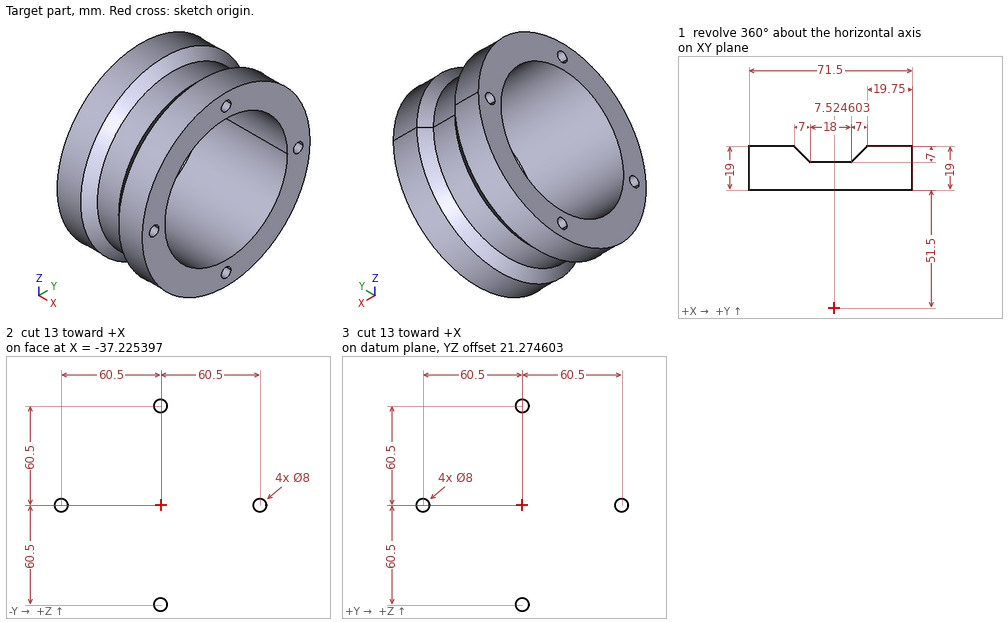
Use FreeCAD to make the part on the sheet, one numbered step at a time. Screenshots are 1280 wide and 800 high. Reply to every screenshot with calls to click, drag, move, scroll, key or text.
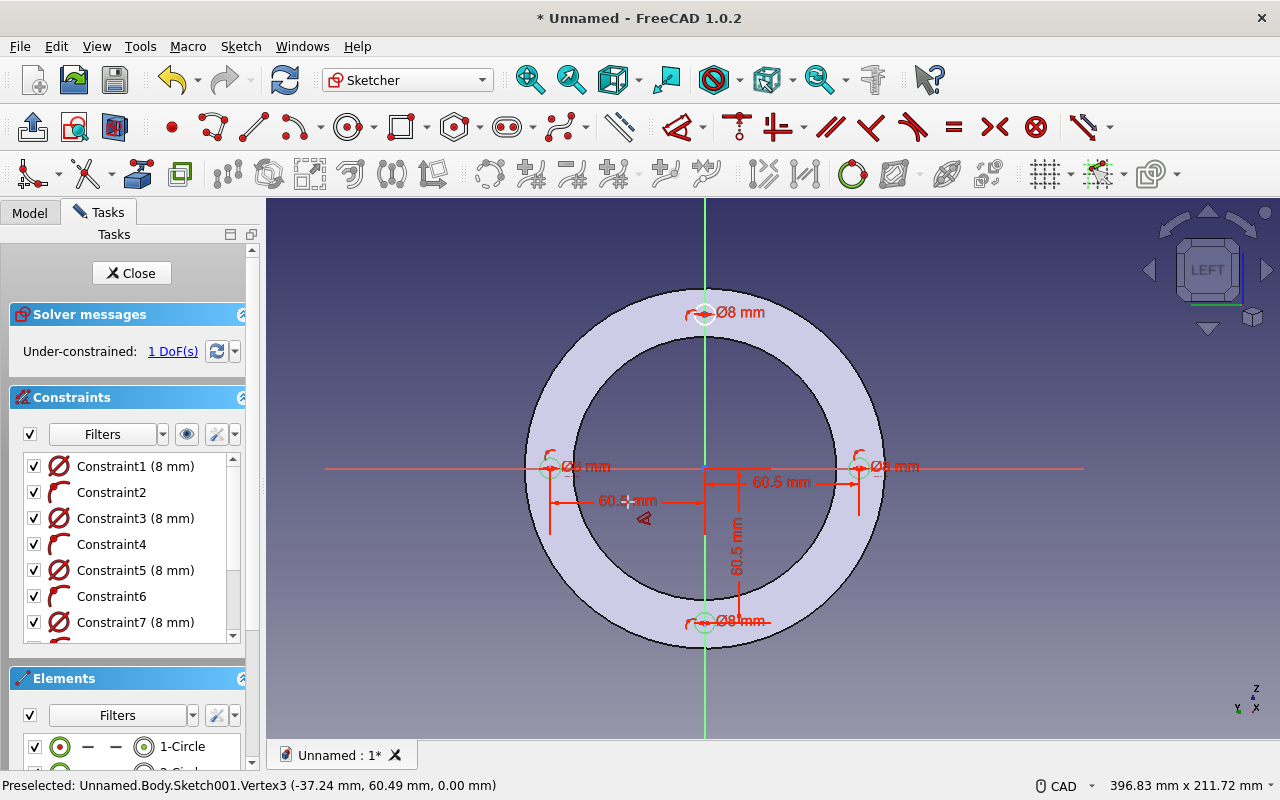
click(705, 314)
click(739, 391)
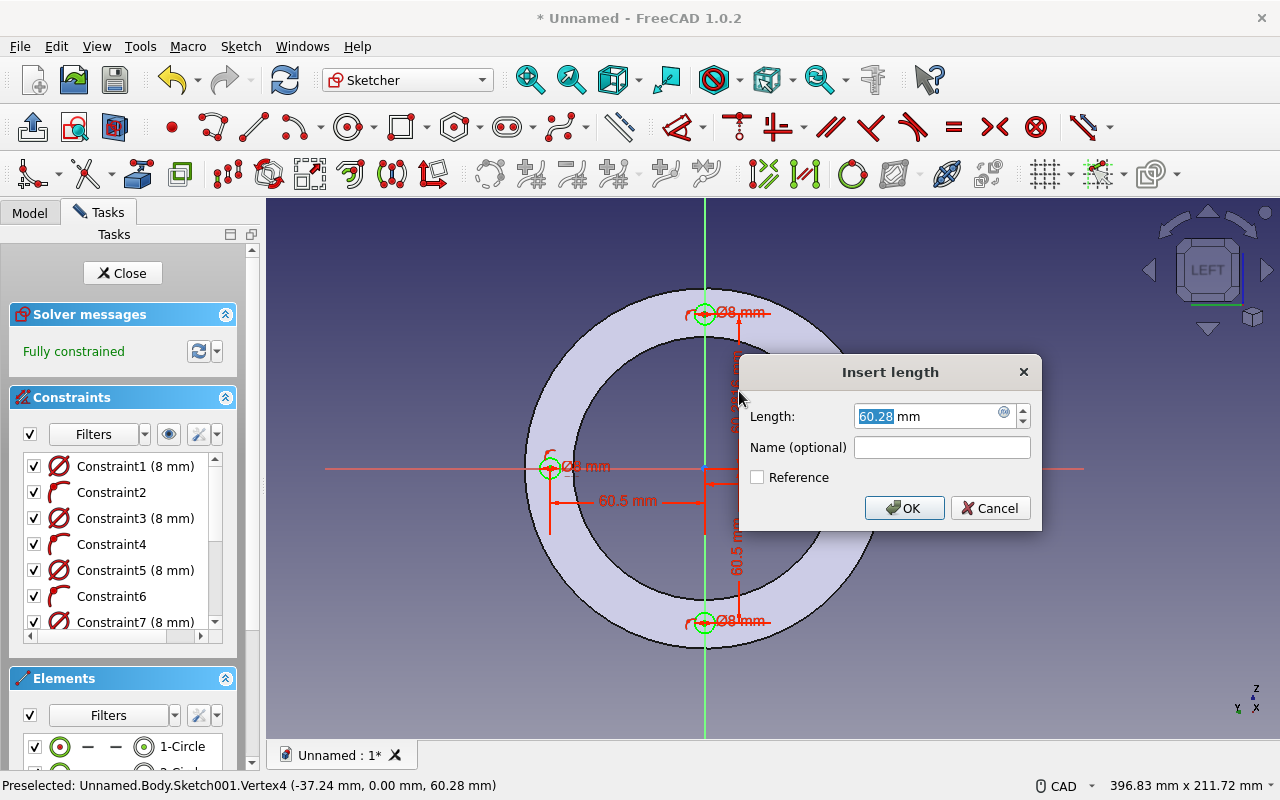
text(60.5)
key(Return)
key(Escape)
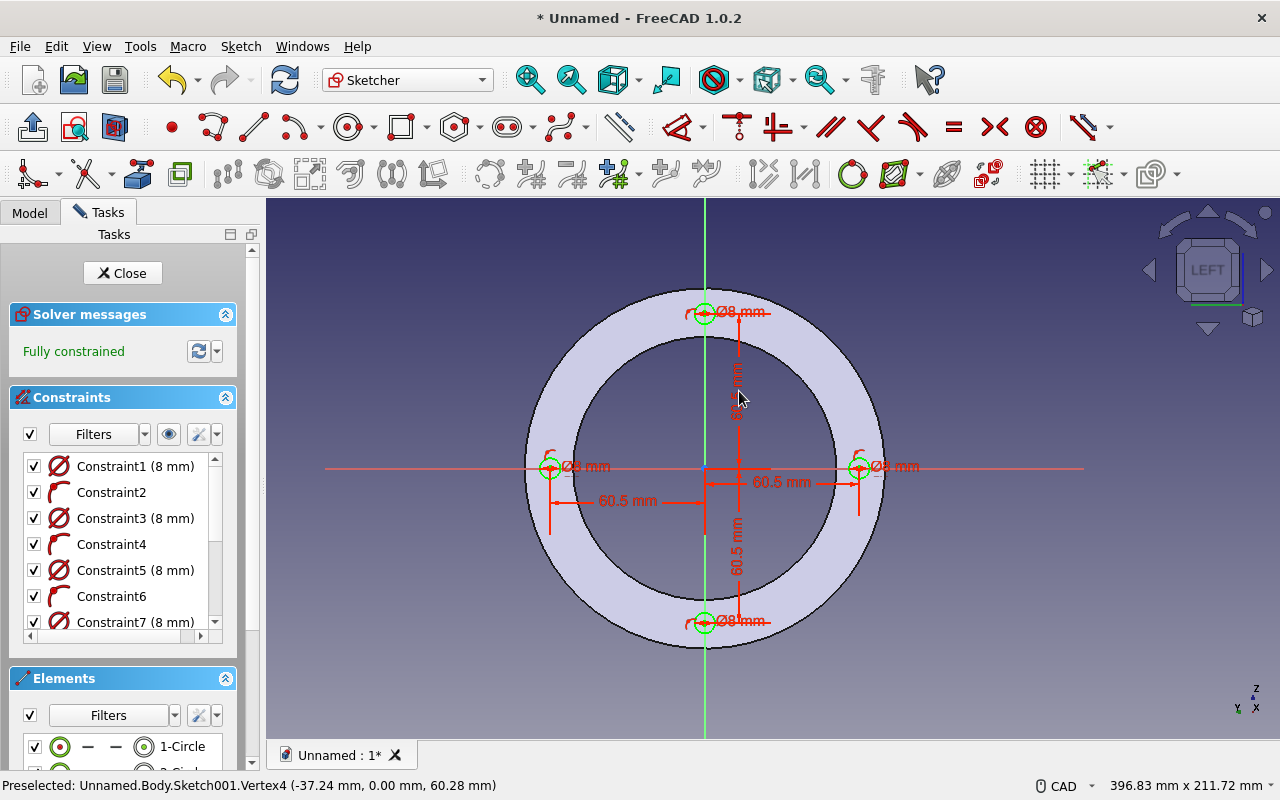
click(123, 273)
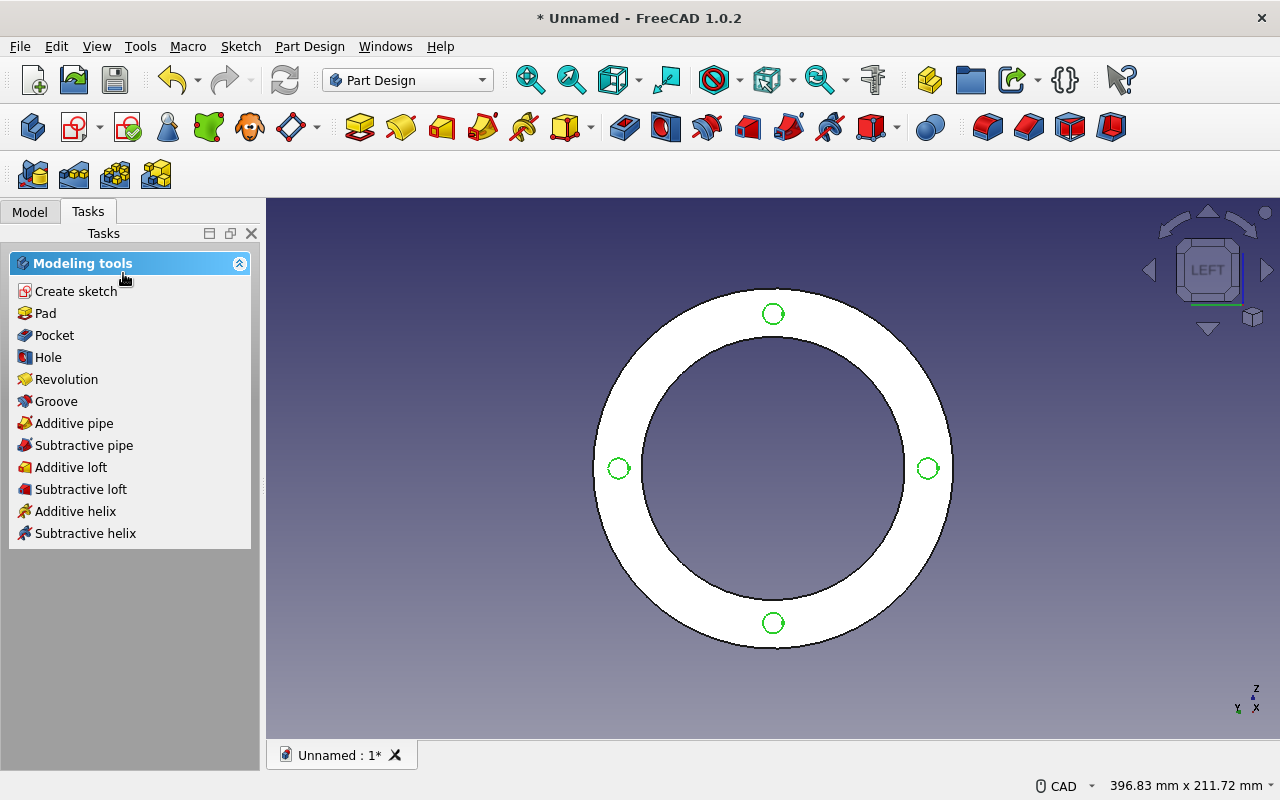
click(625, 128)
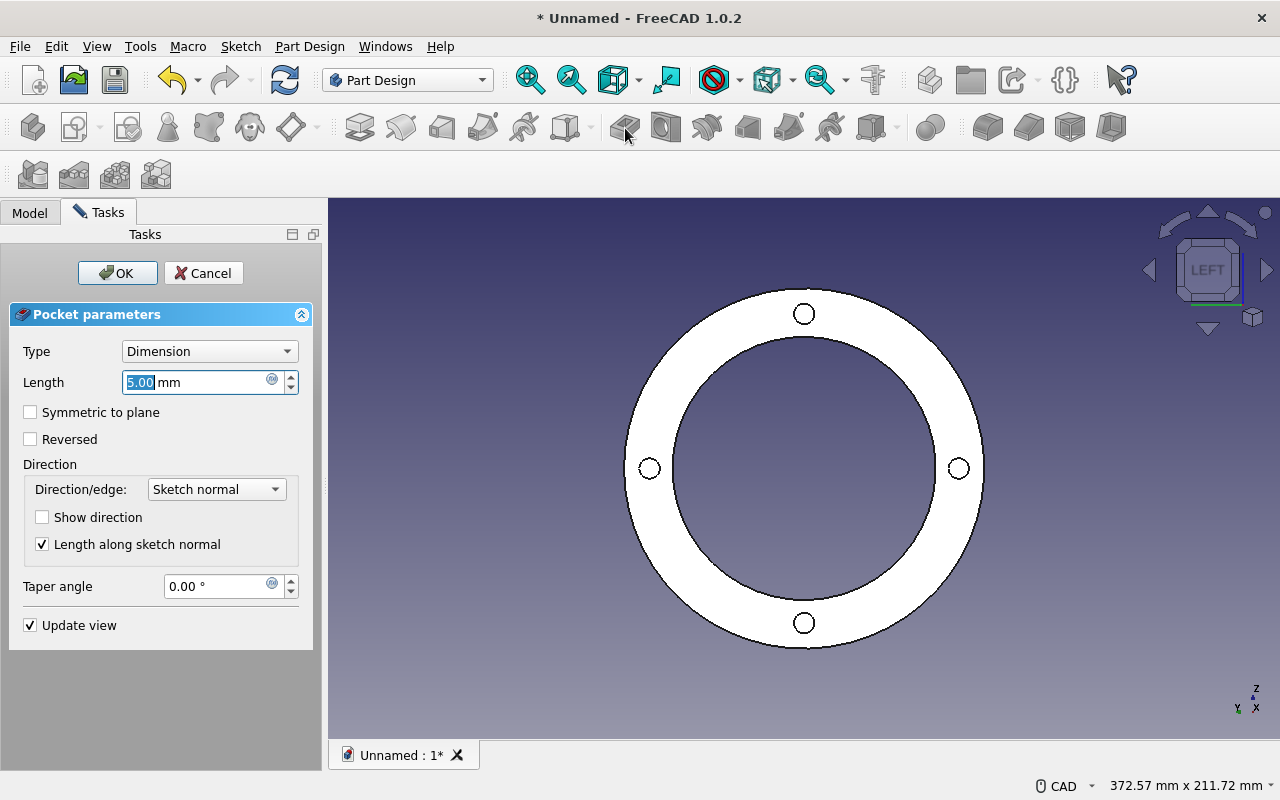
text(13)
key(Tab)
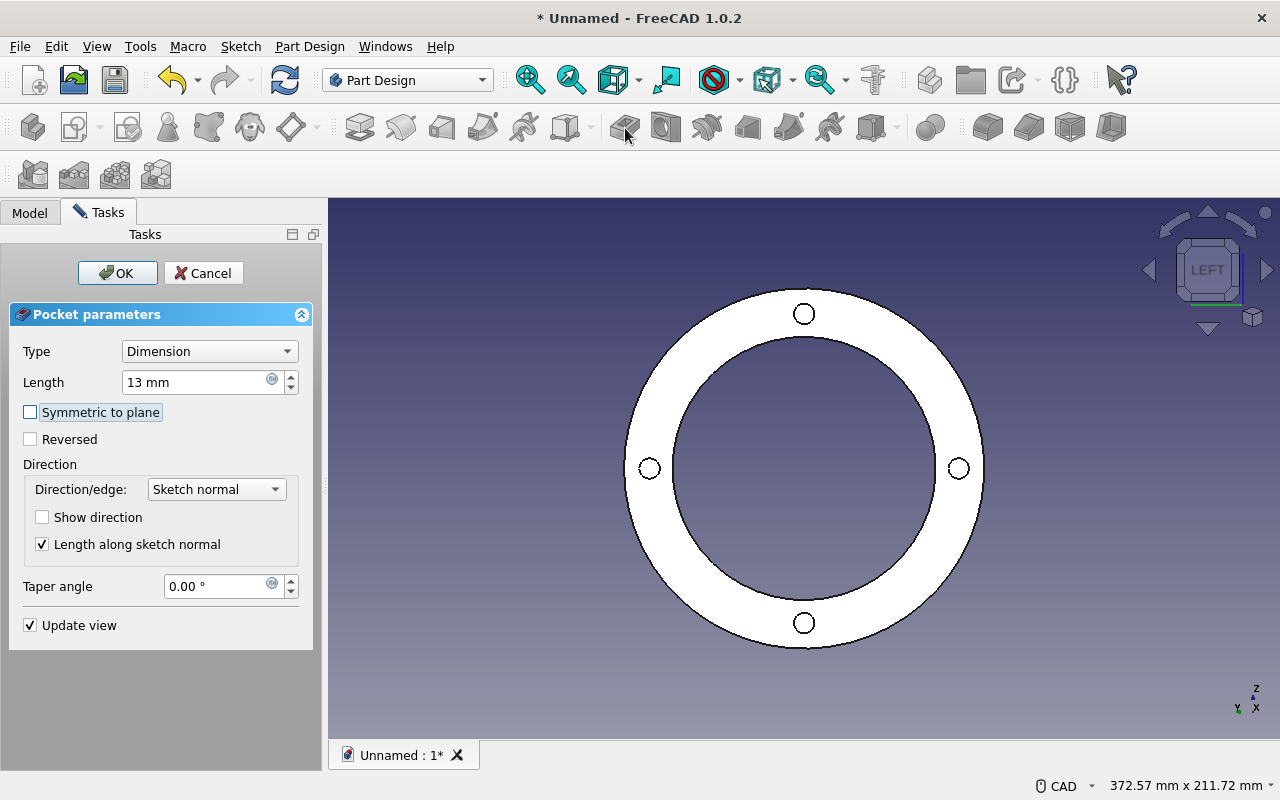
click(118, 273)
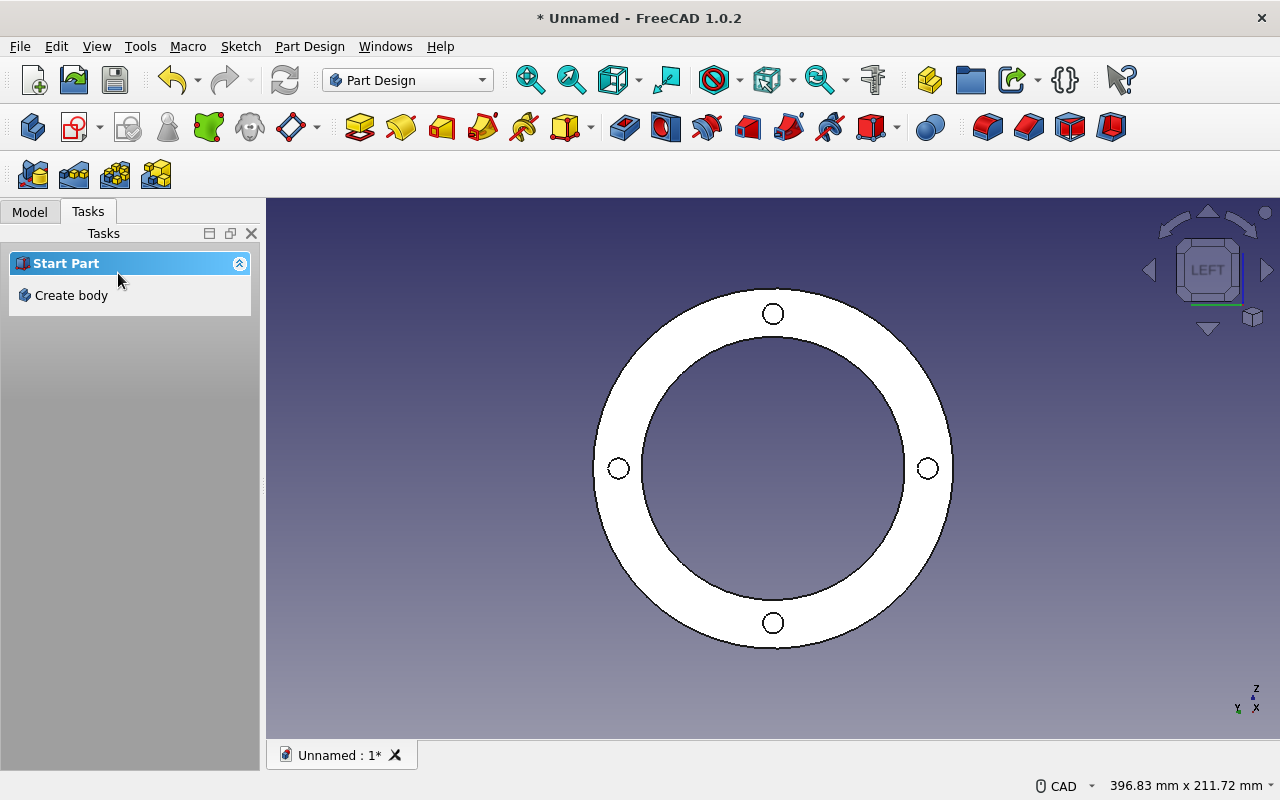
click(30, 212)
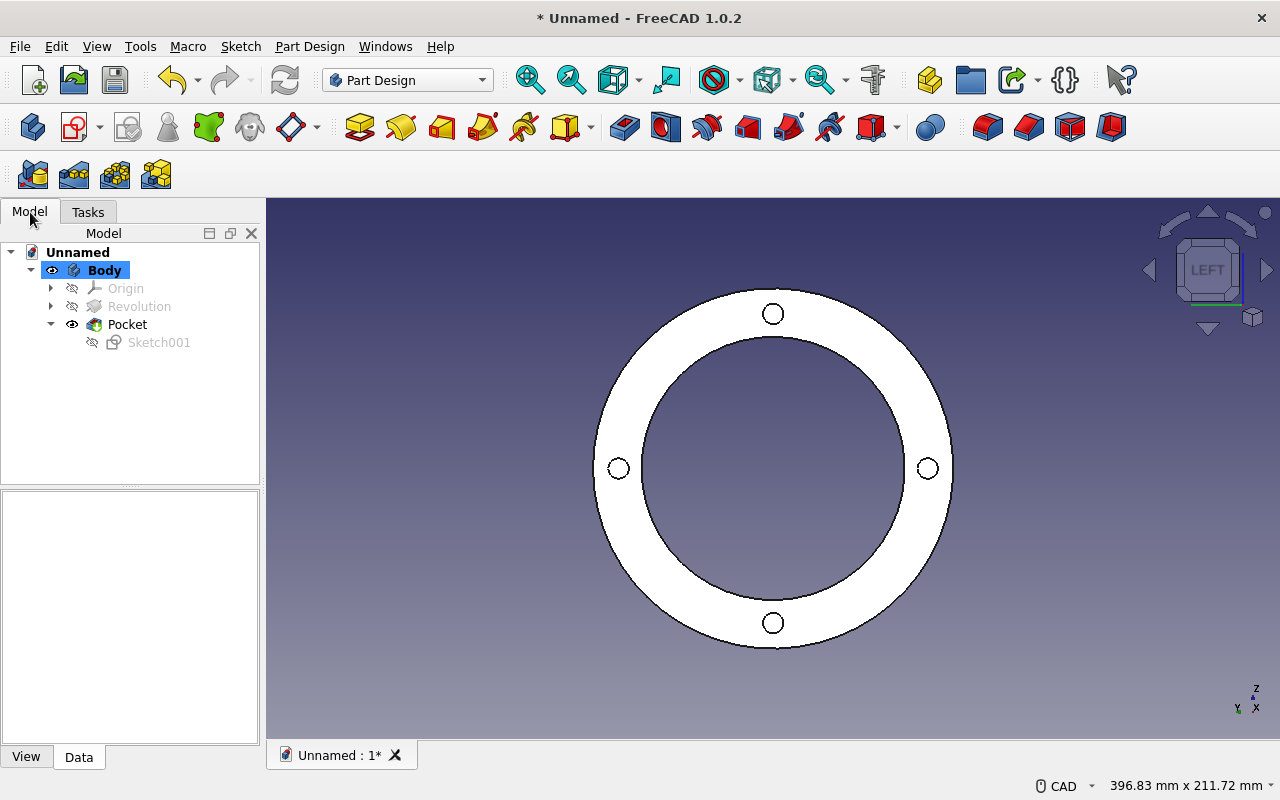
click(51, 288)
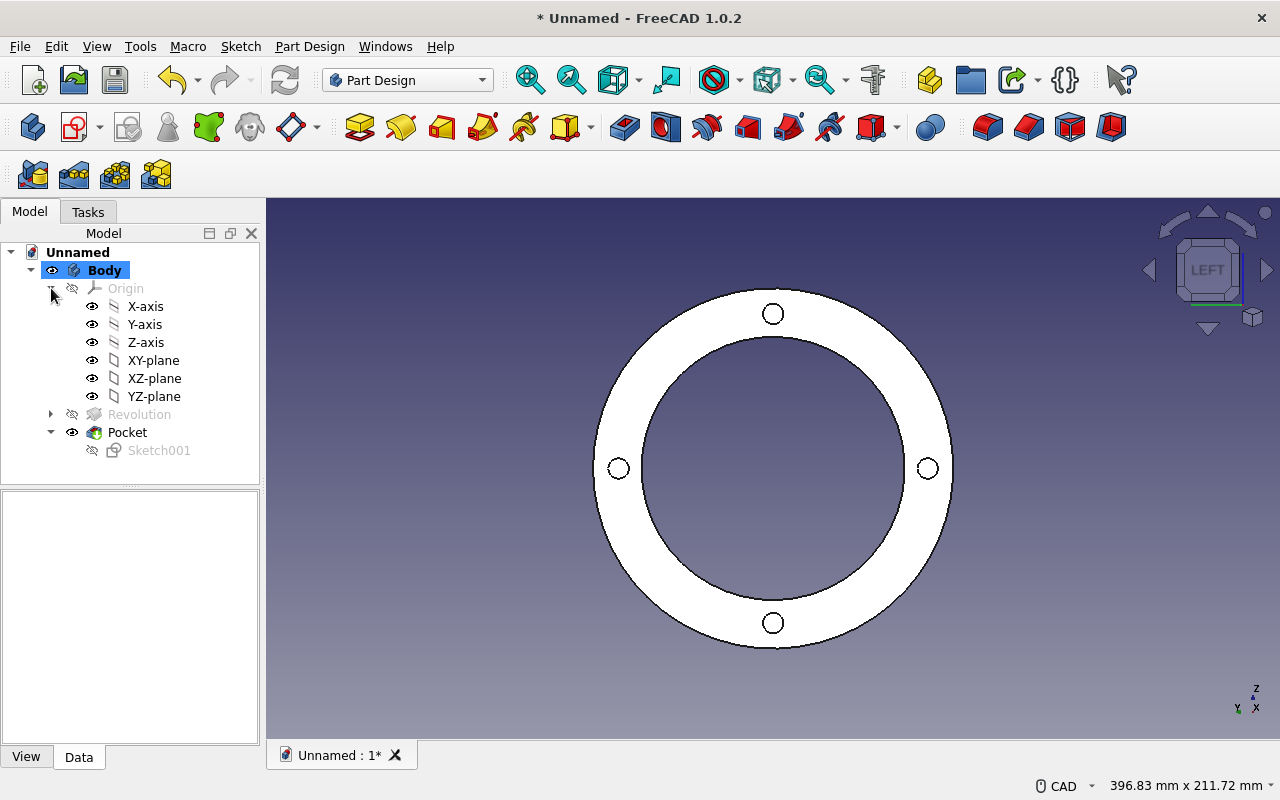
click(137, 396)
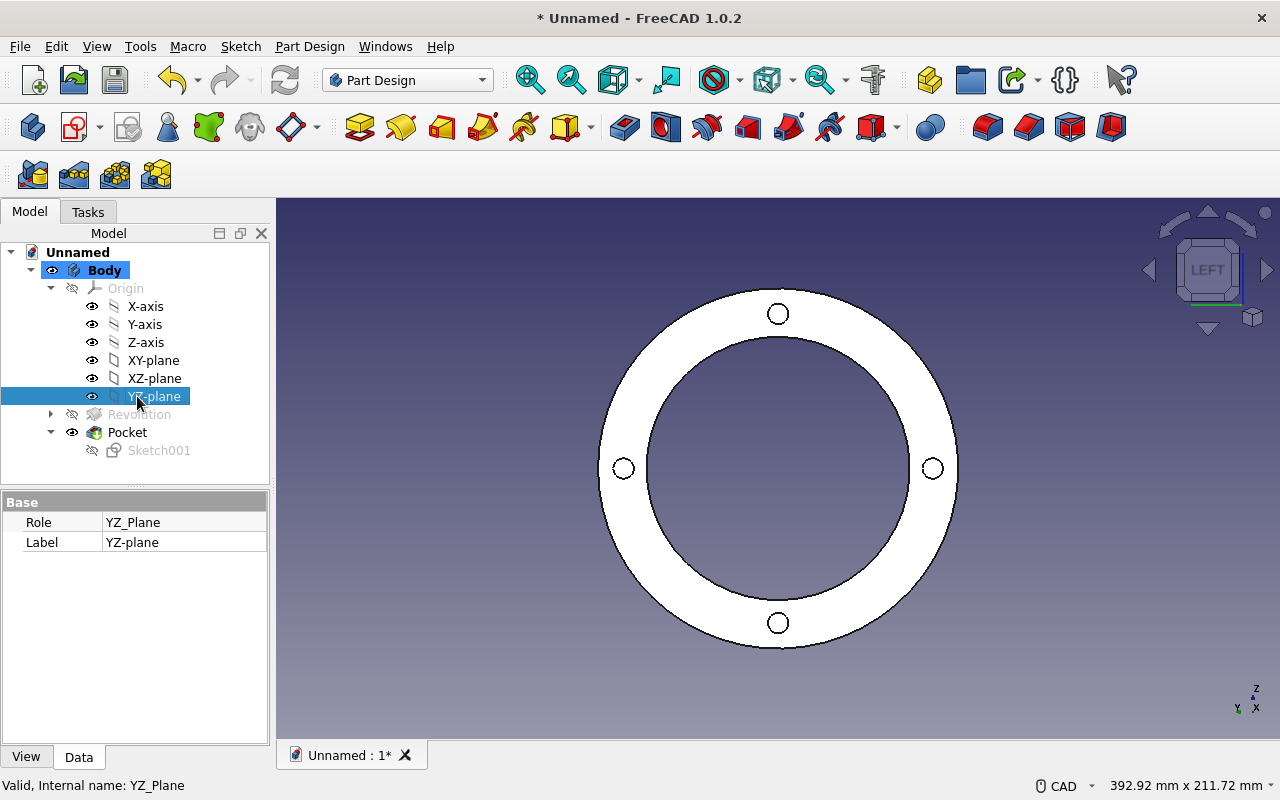
click(290, 128)